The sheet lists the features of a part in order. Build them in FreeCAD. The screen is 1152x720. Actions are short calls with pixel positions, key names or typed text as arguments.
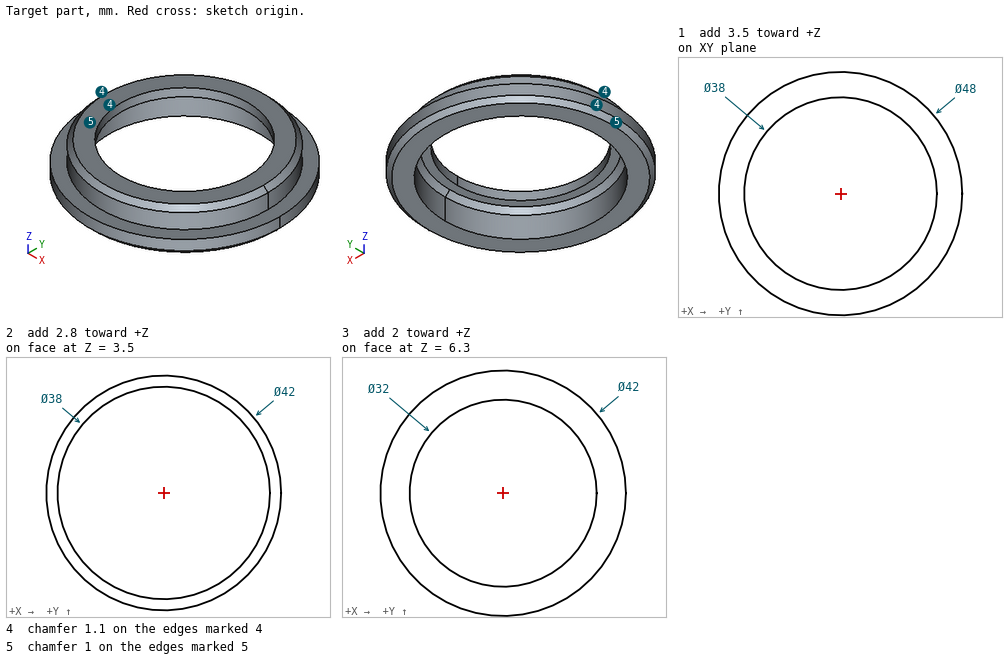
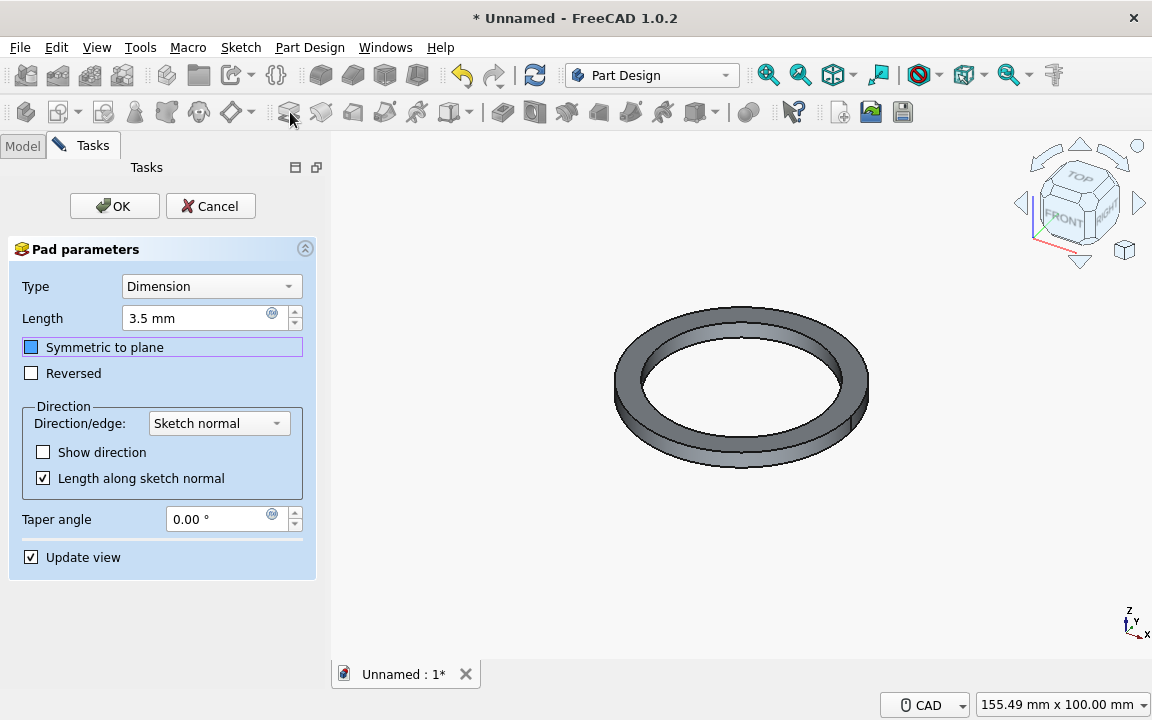
click(115, 206)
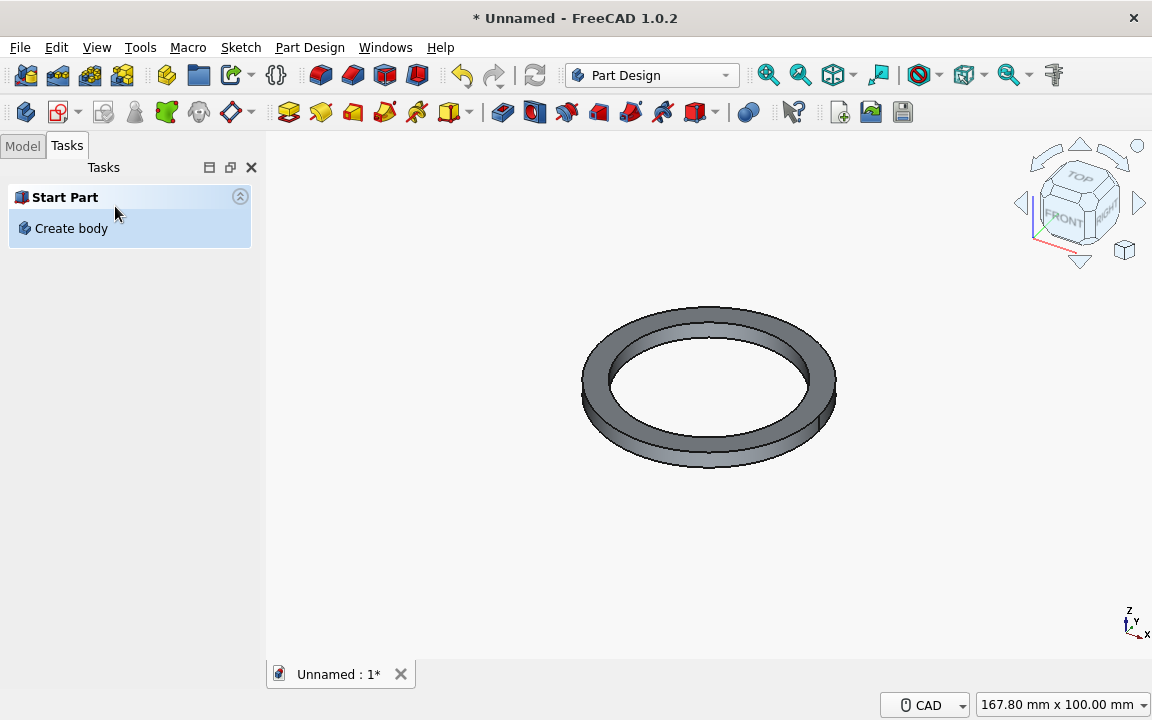
click(770, 76)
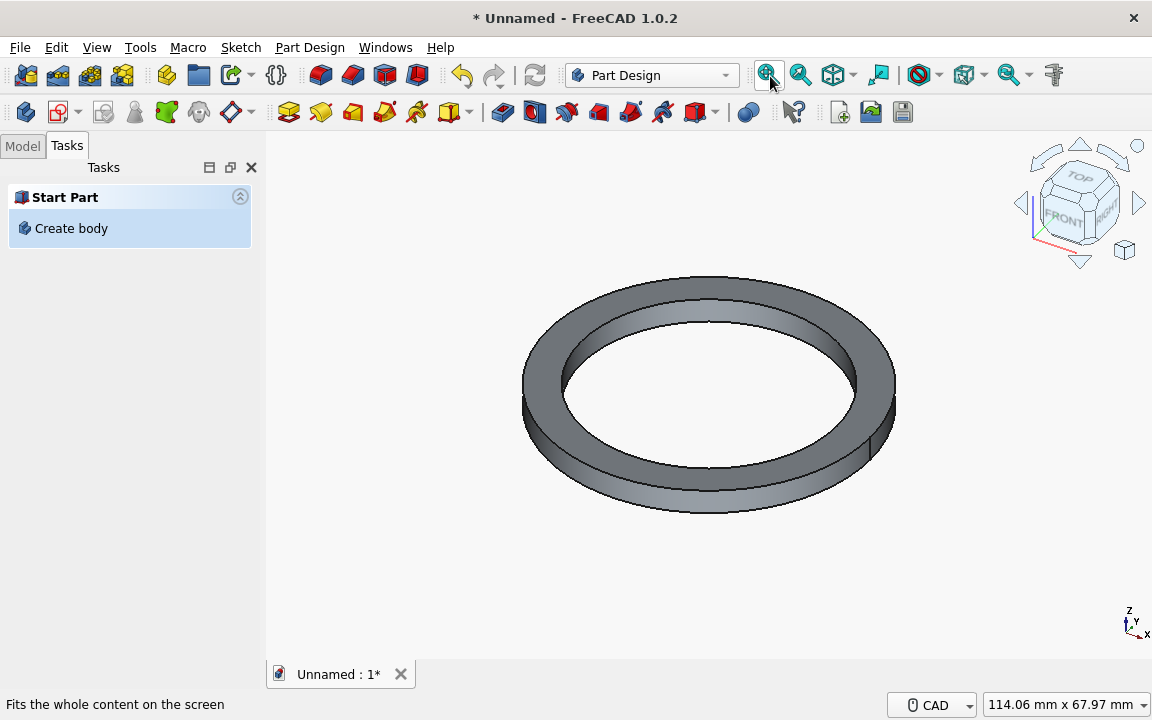
click(821, 455)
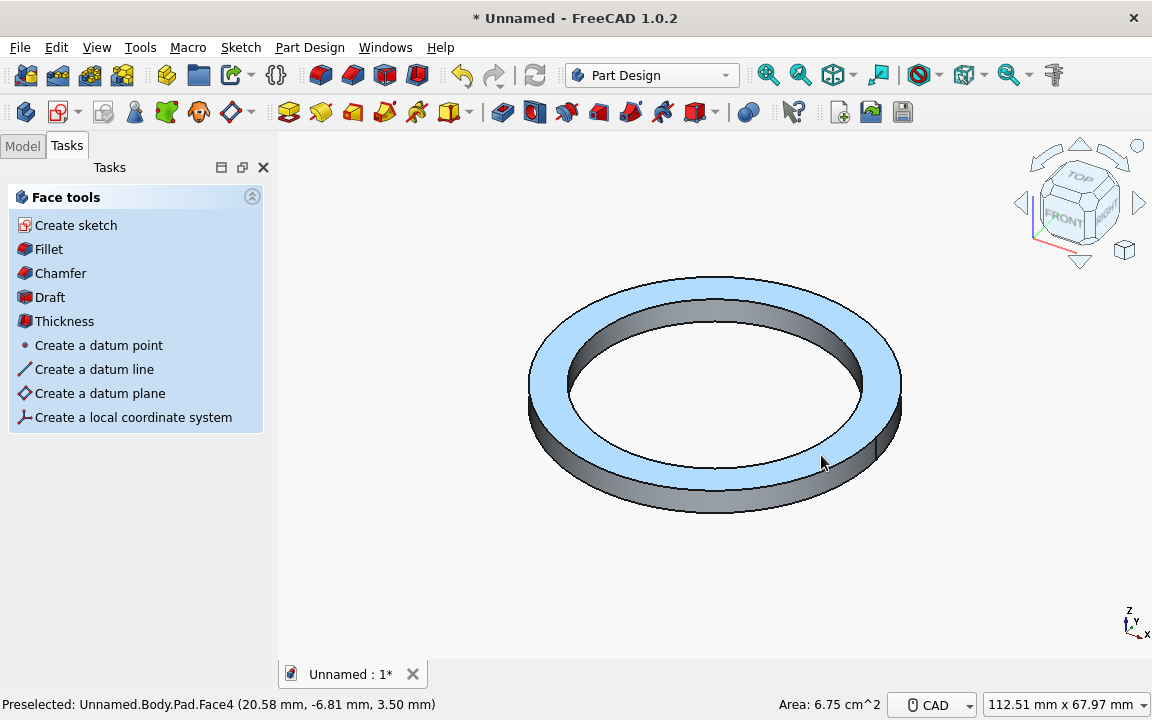
click(58, 112)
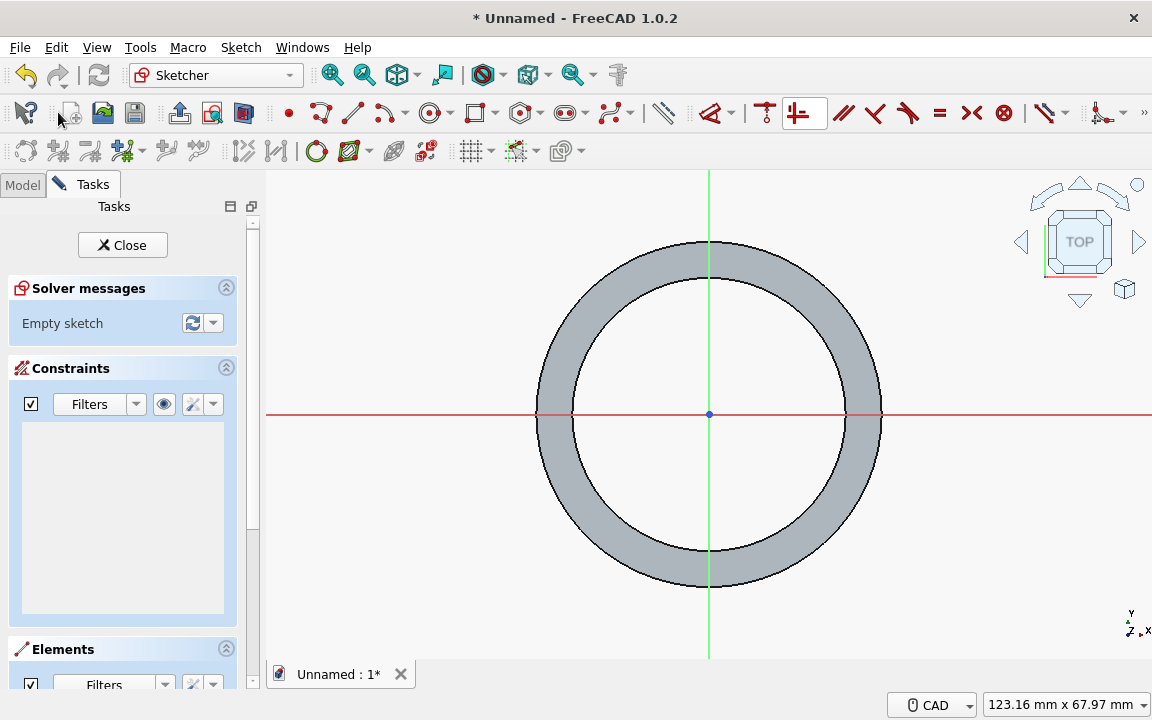
click(430, 114)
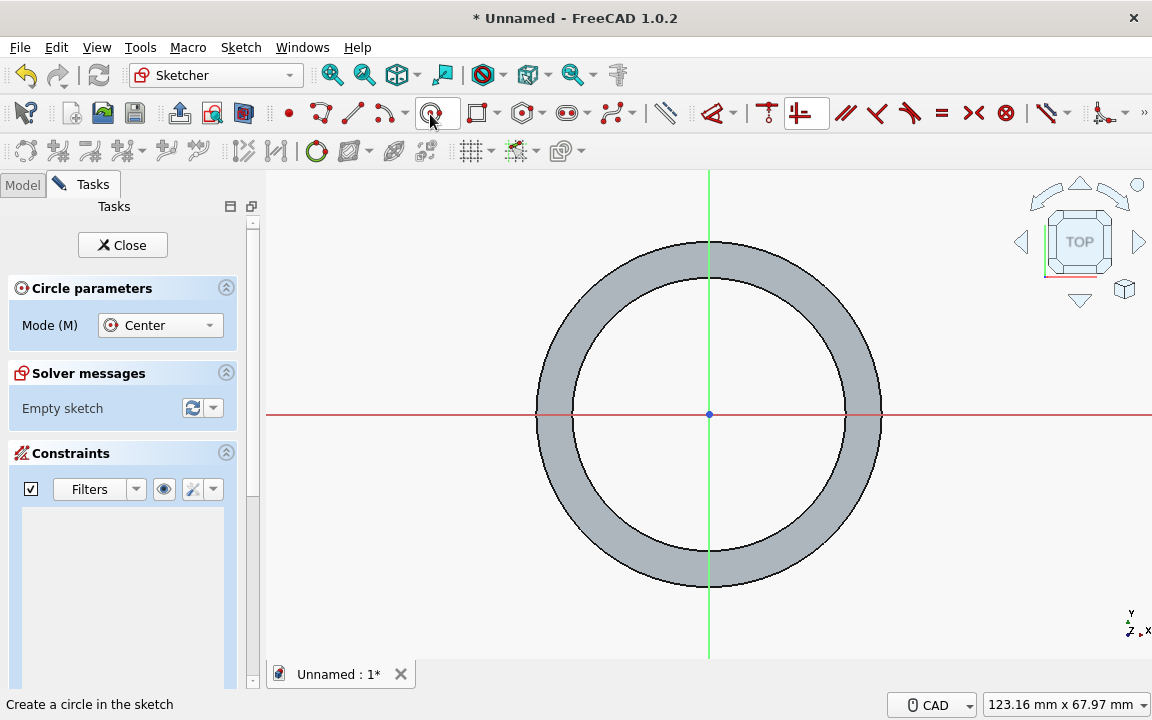
click(709, 414)
move(816, 308)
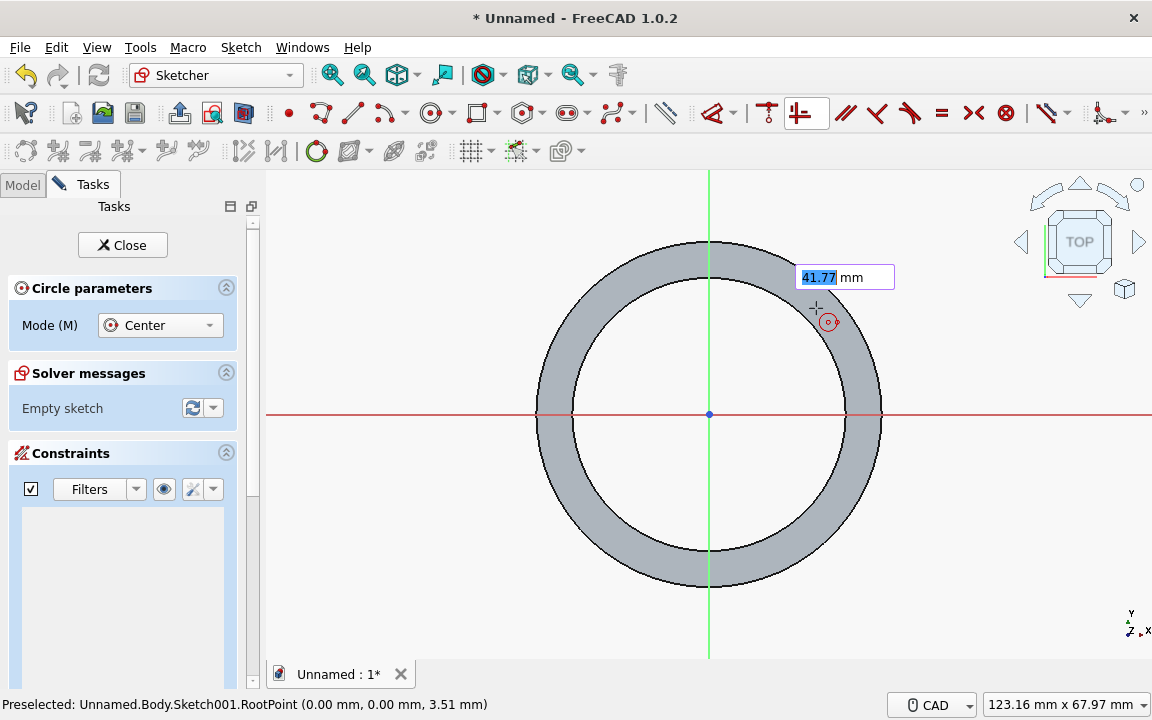
text(42)
key(Return)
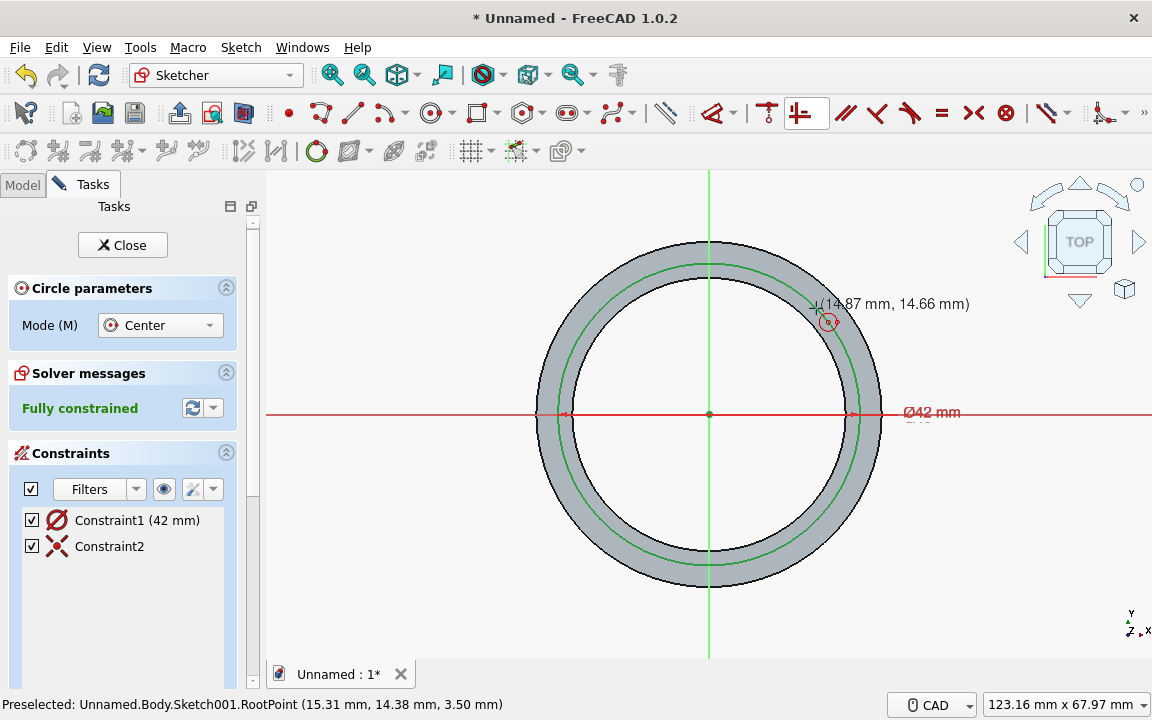
click(709, 414)
move(806, 318)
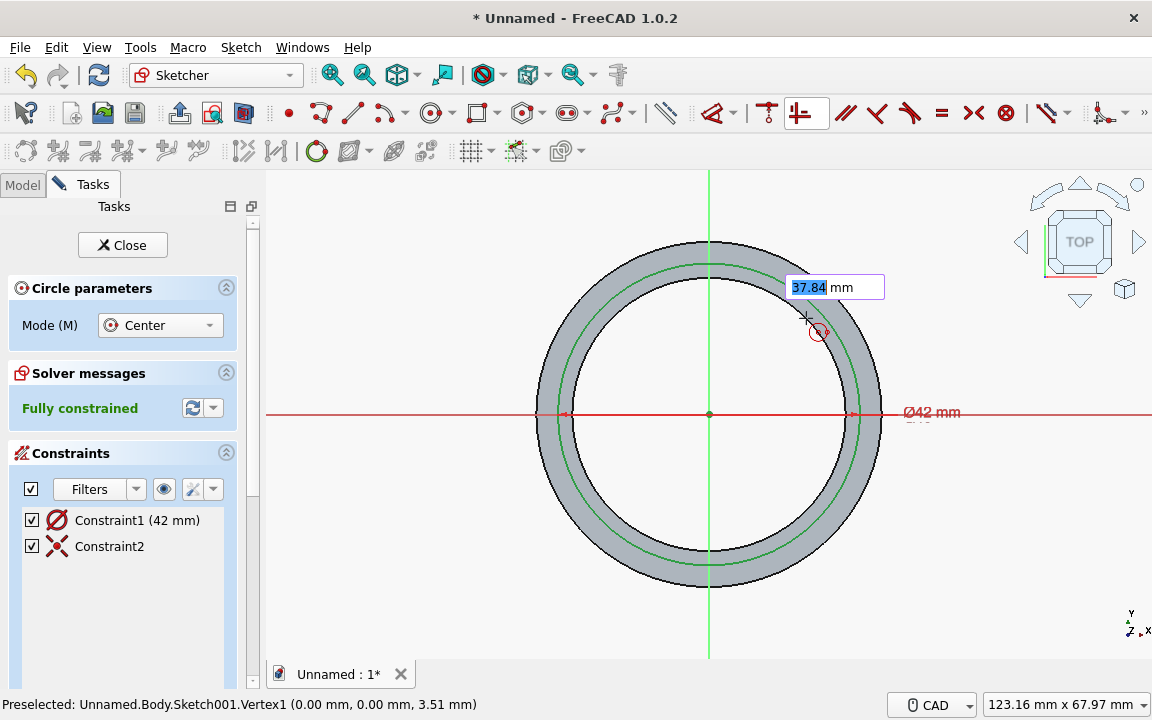
text(38)
key(Return)
key(Escape)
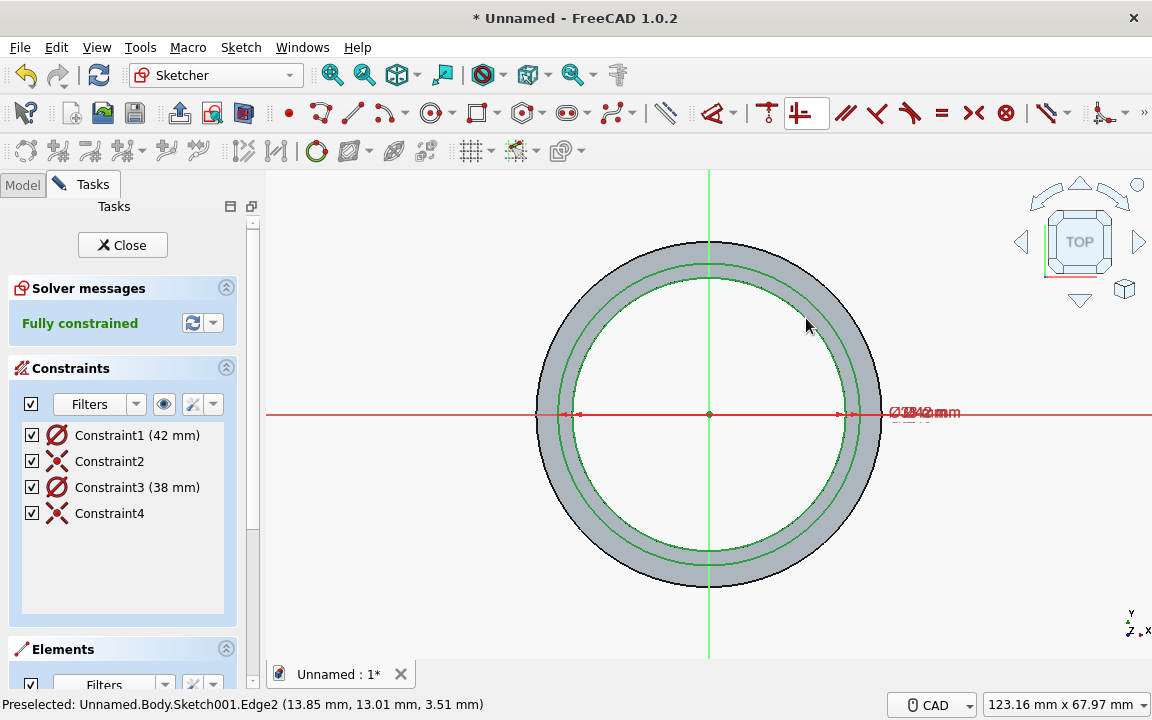
click(123, 245)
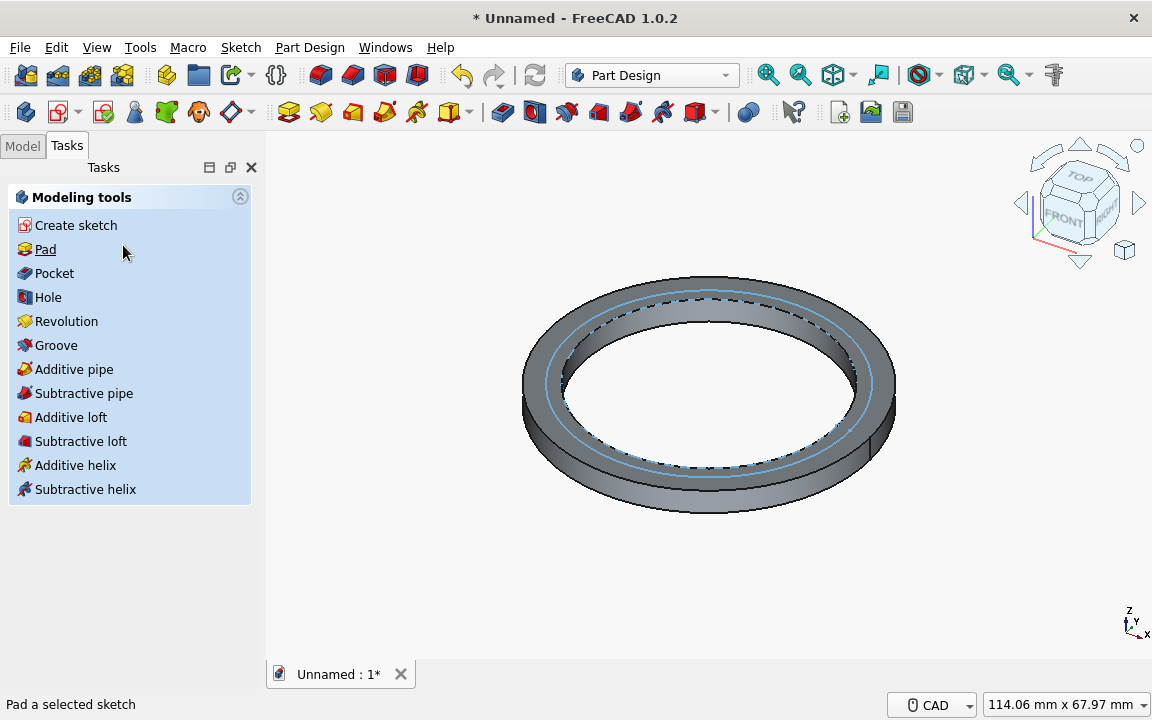
click(290, 112)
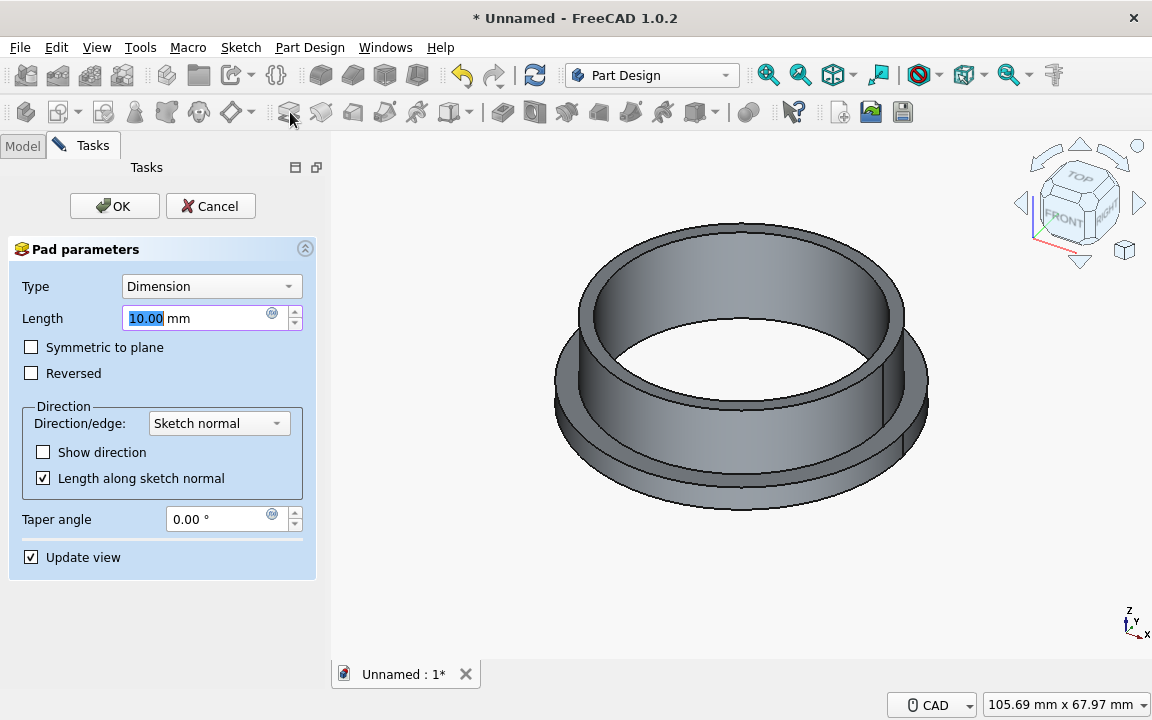
text(2.8)
key(Tab)